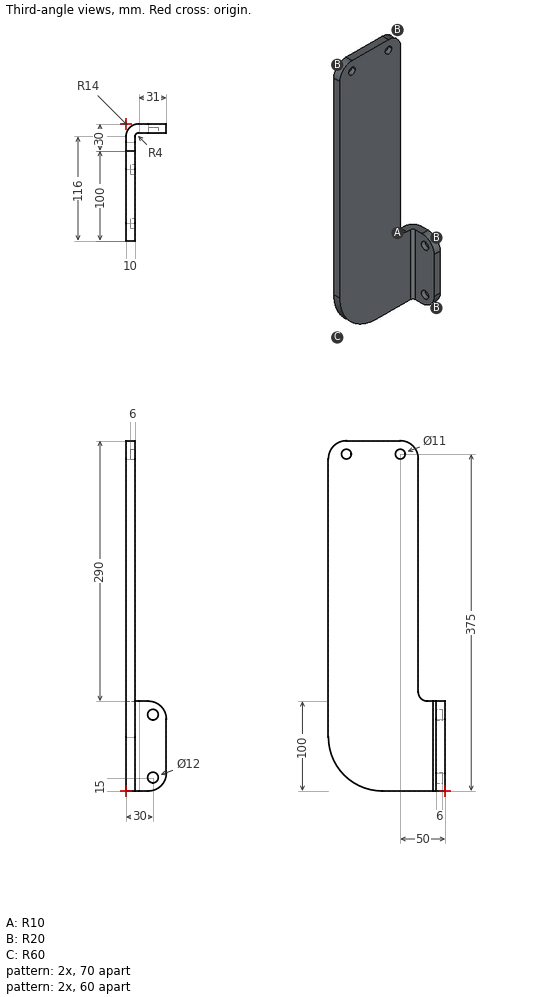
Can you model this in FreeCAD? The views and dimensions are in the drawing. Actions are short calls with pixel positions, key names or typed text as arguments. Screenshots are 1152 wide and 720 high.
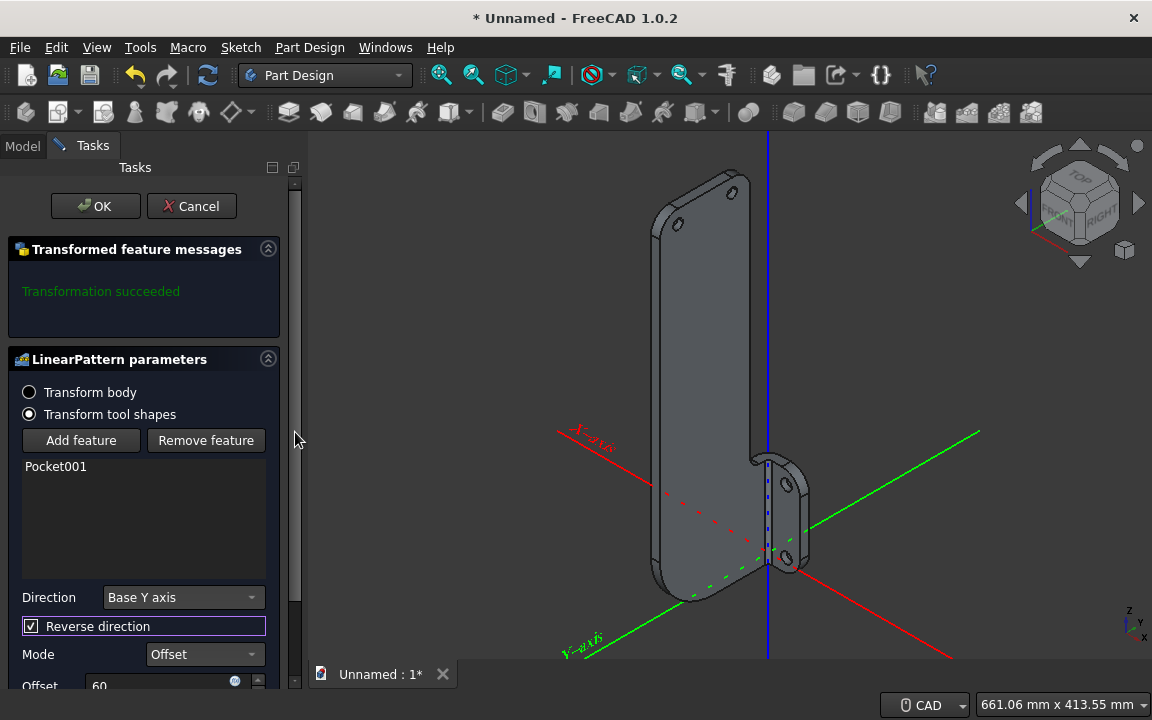
click(96, 206)